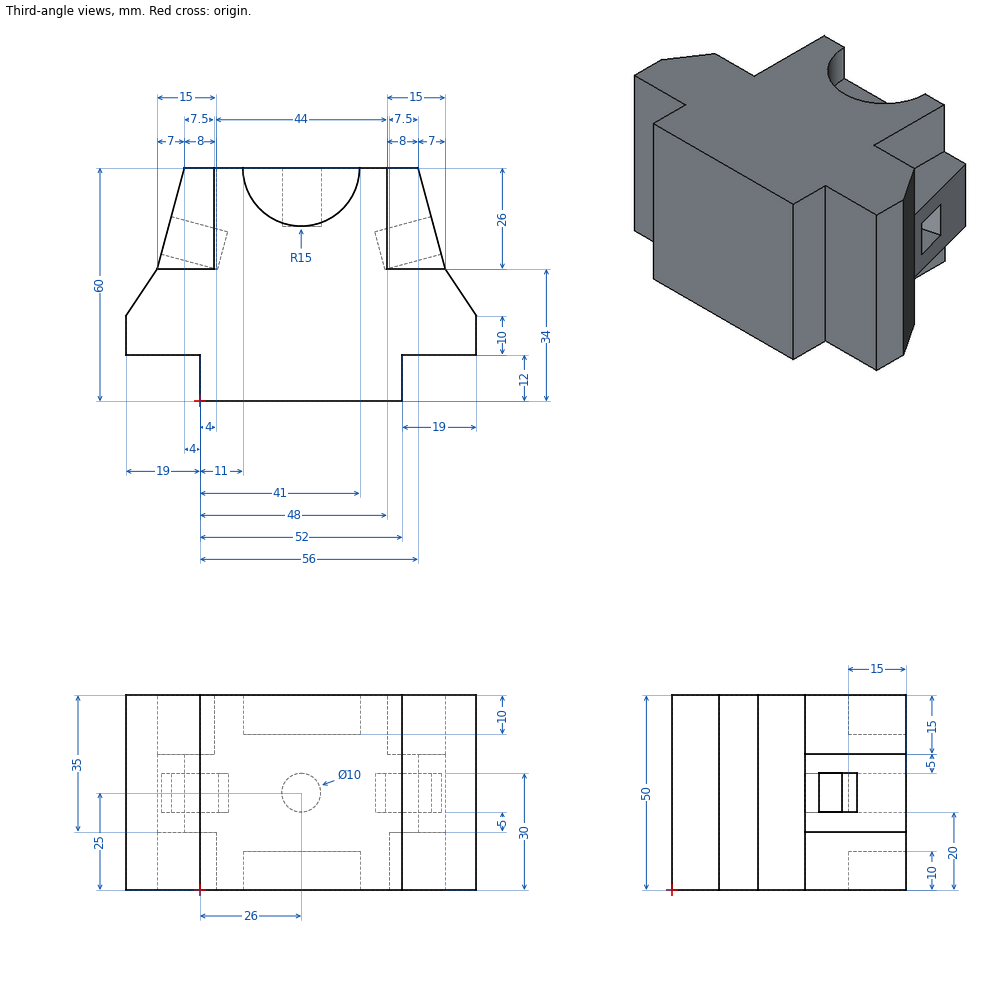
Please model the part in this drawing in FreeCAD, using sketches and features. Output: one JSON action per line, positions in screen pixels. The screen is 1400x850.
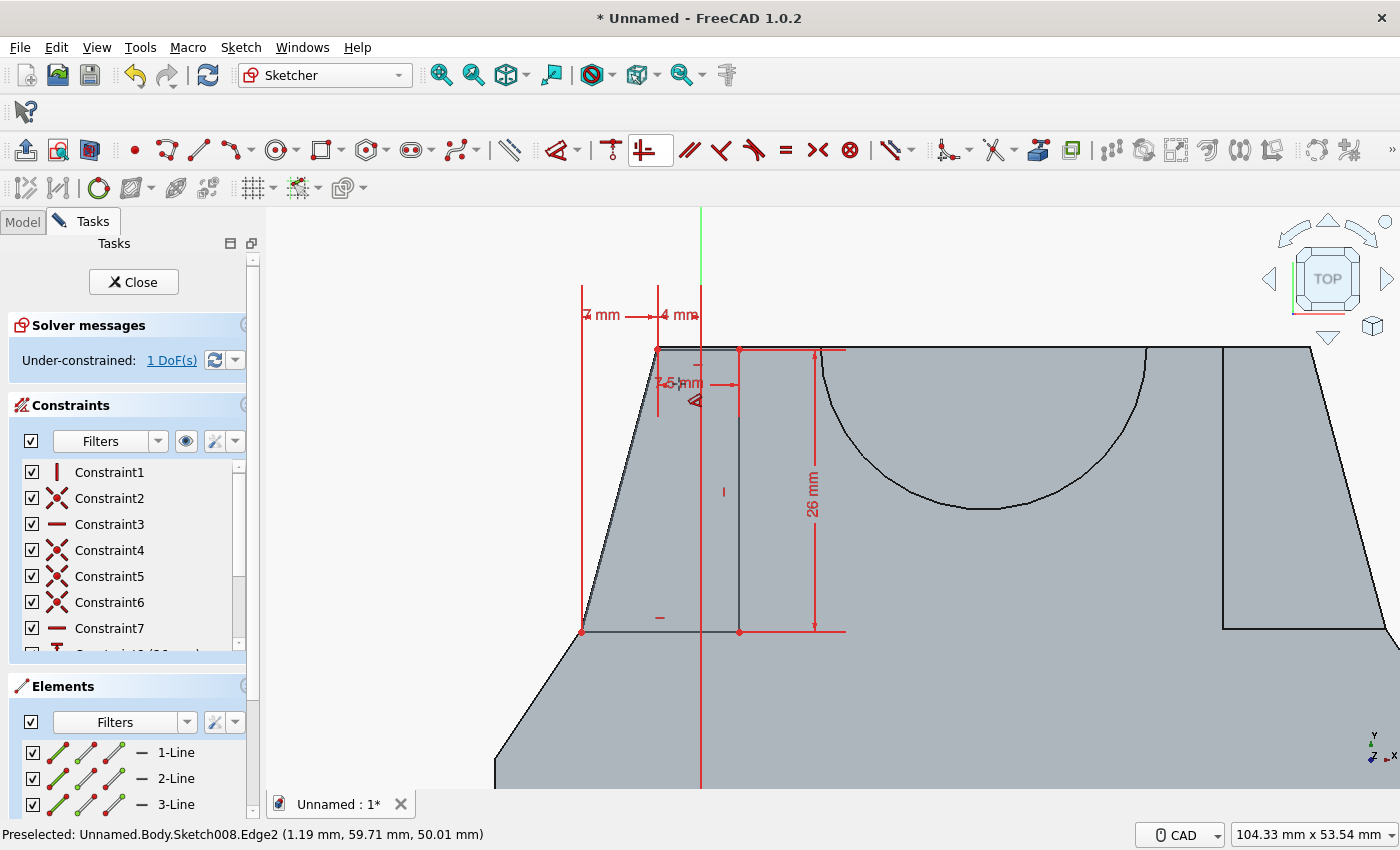
{"action": "left_click", "coordinate": [739, 632]}
{"action": "left_click", "coordinate": [773, 697]}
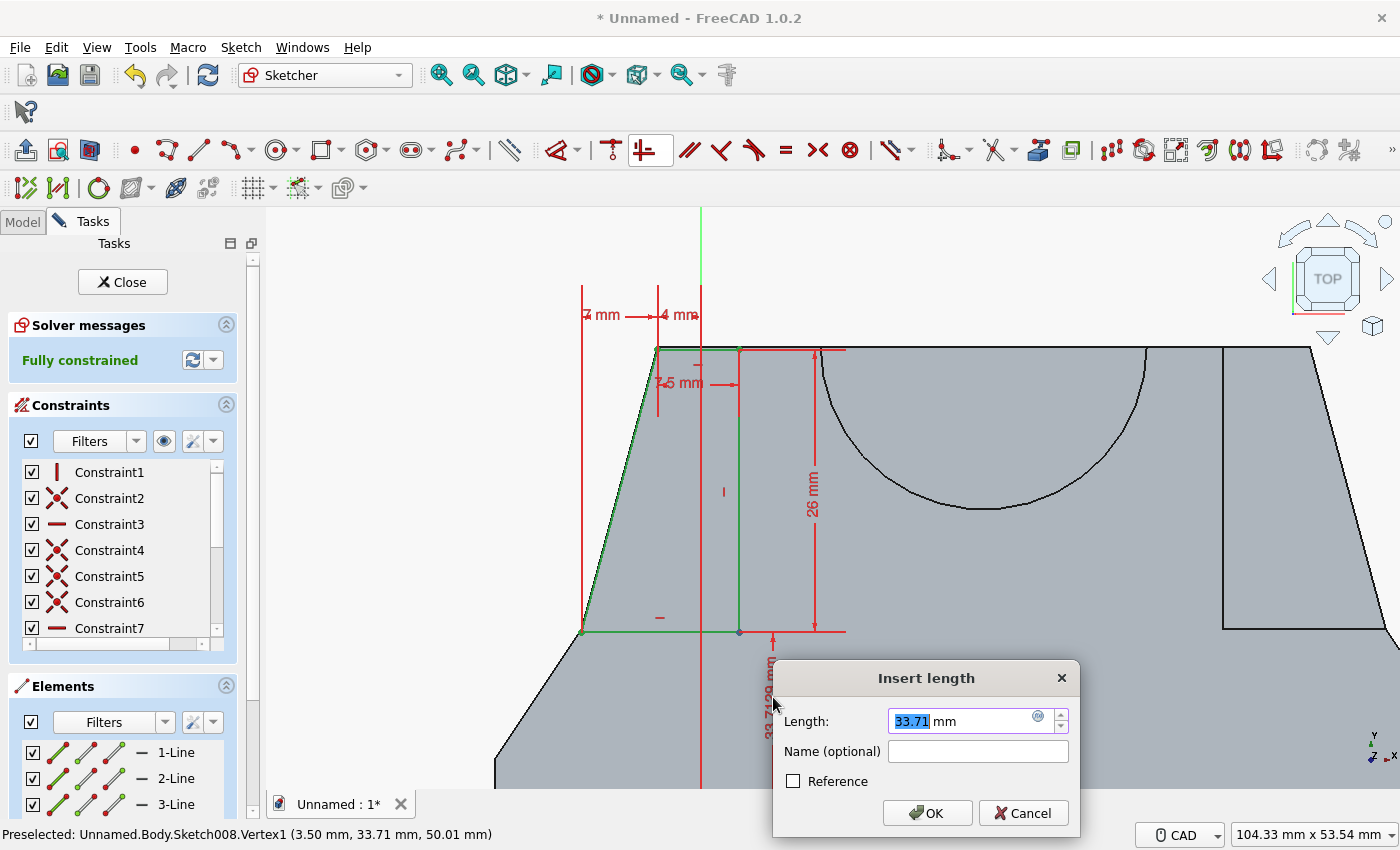
{"action": "type", "text": "34"}
{"action": "key", "text": "Return"}
{"action": "key", "text": "Escape"}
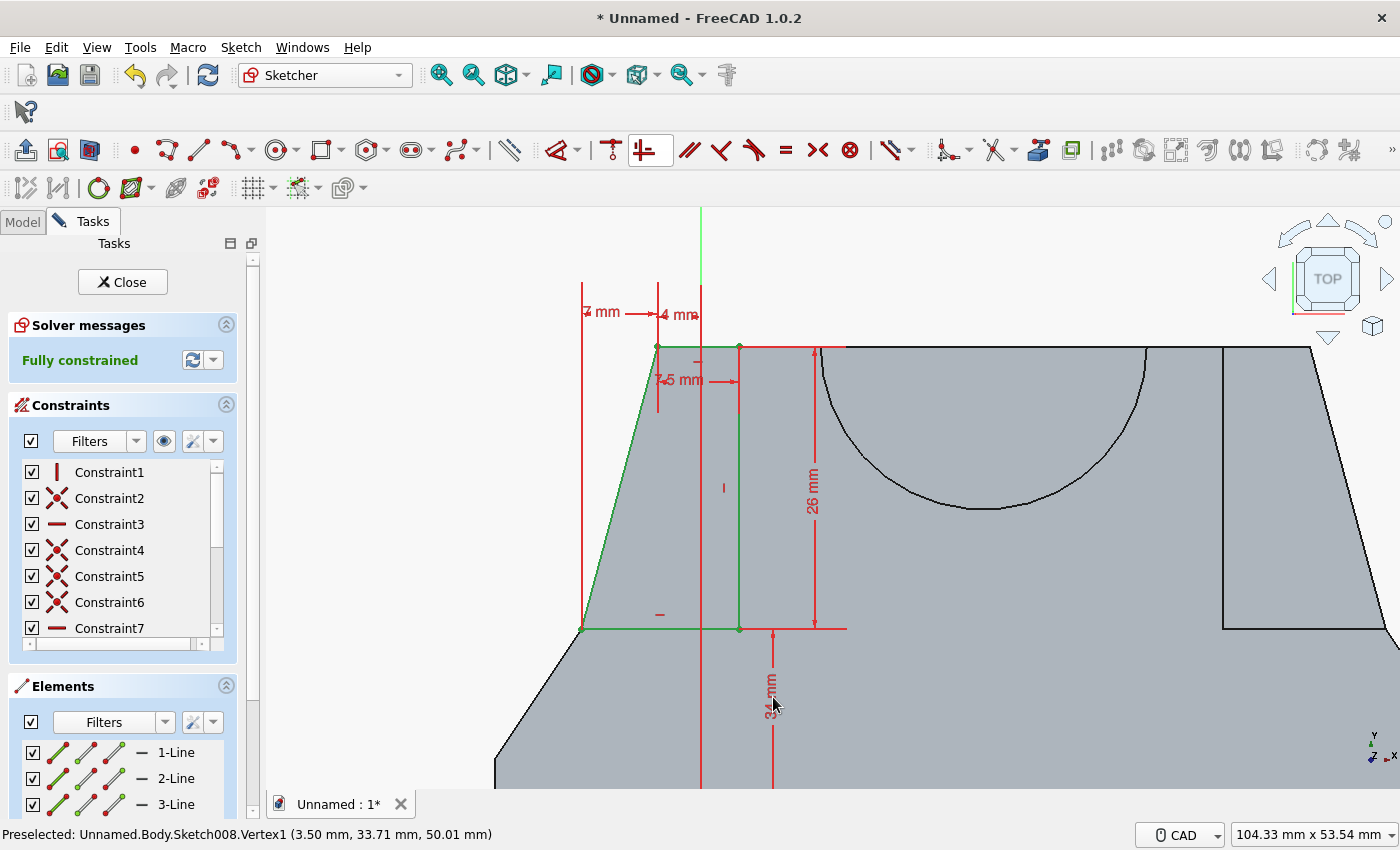
{"action": "left_click", "coordinate": [123, 282]}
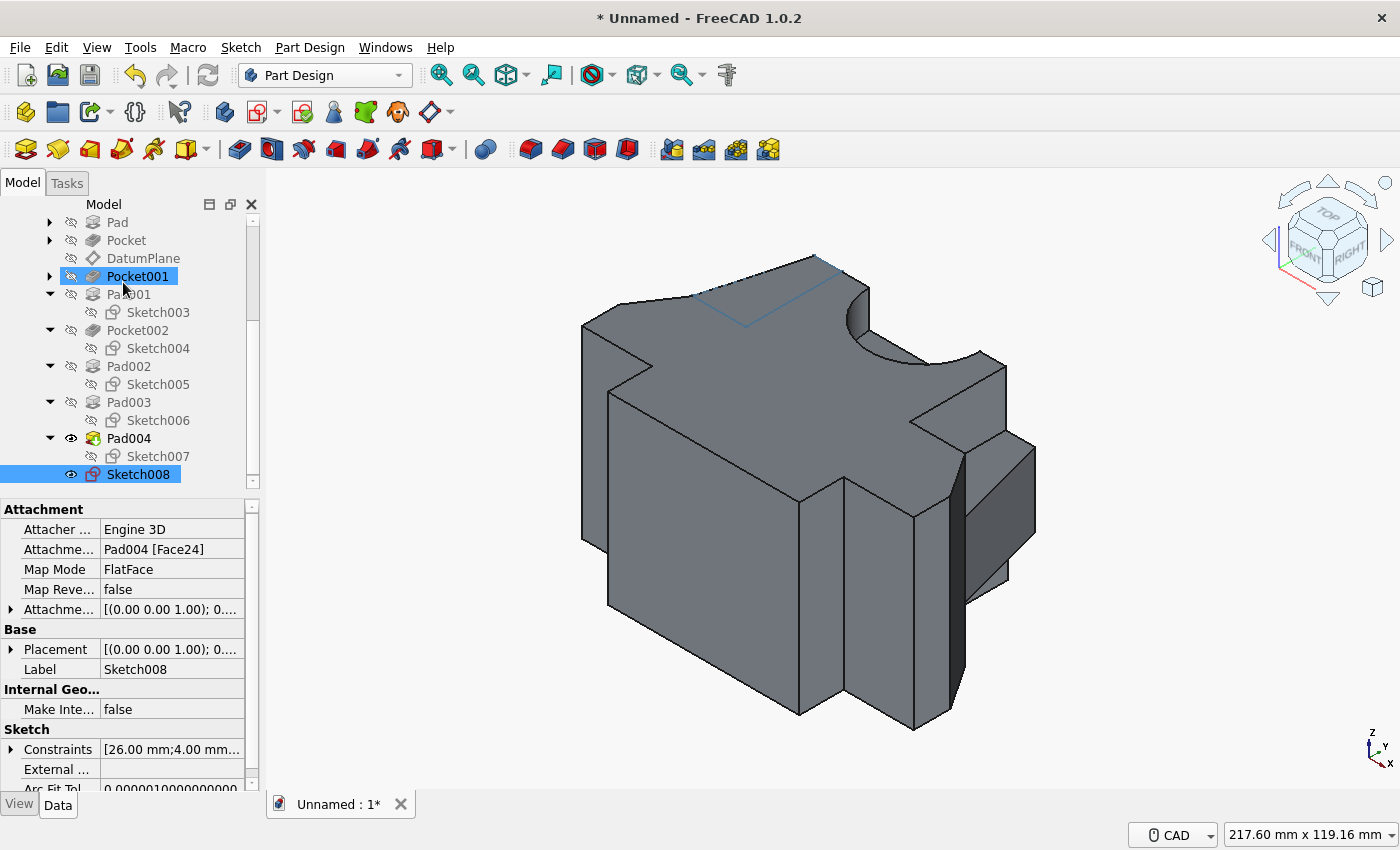
{"action": "left_click", "coordinate": [240, 150]}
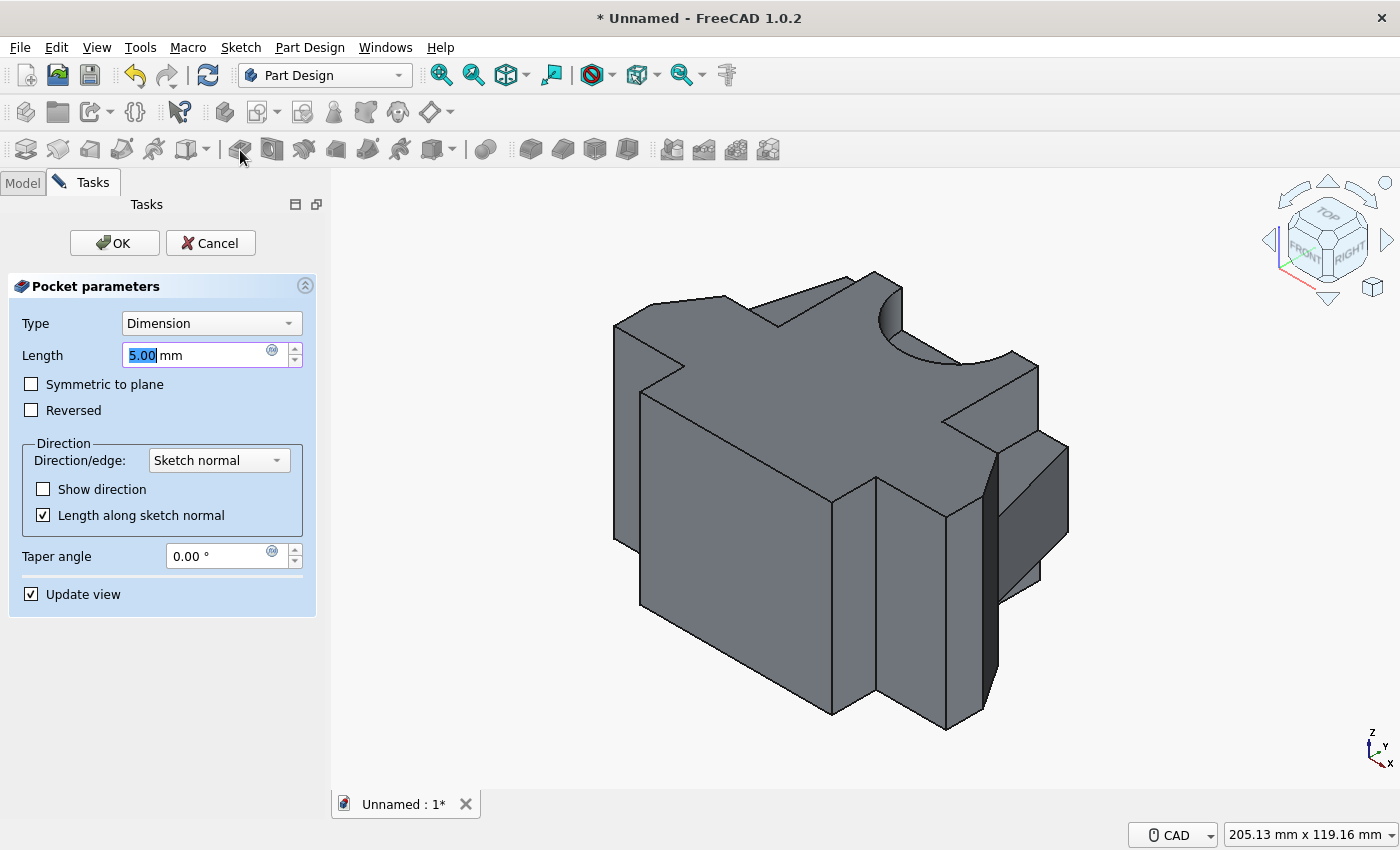
{"action": "type", "text": "15"}
{"action": "key", "text": "Tab"}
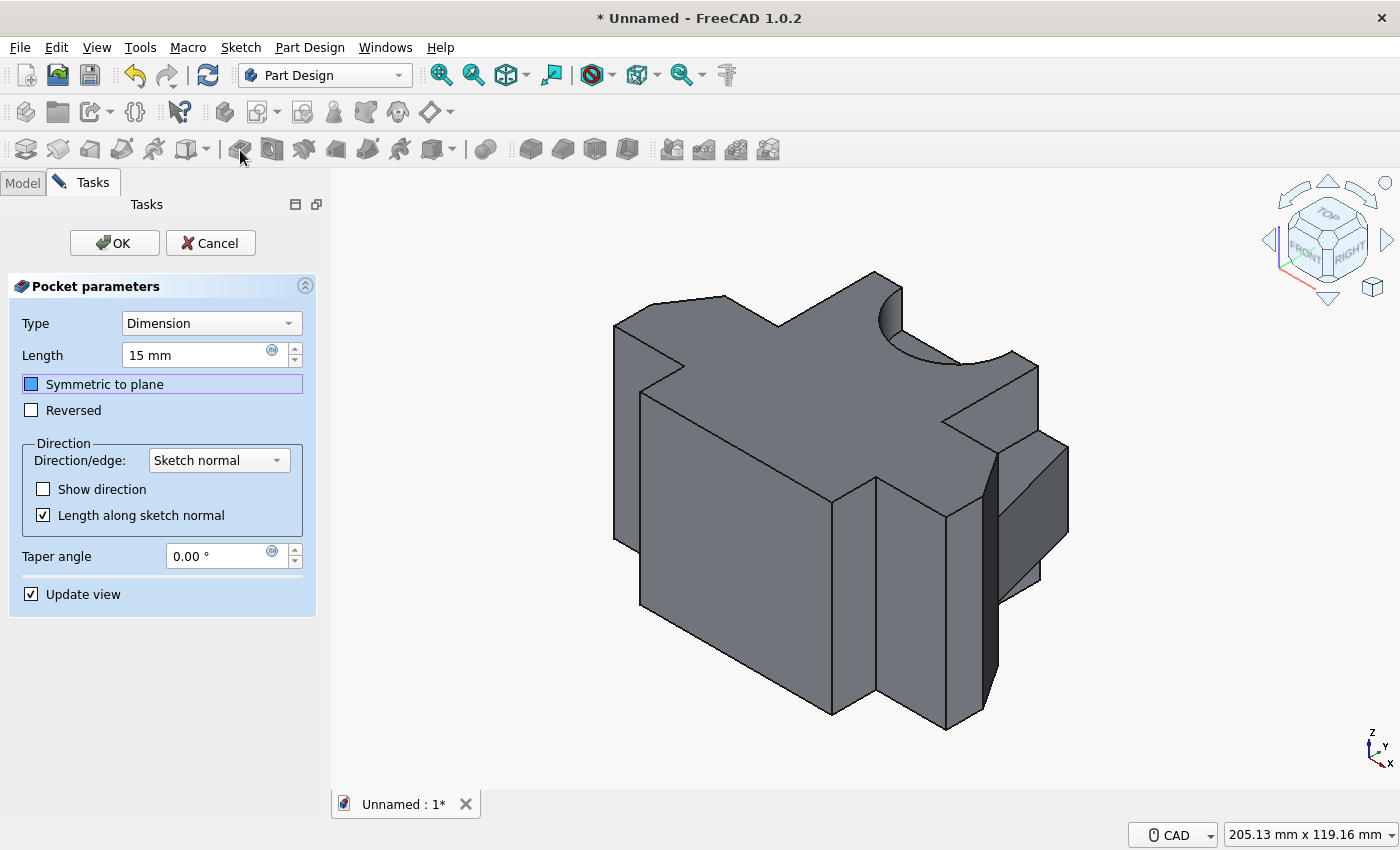
{"action": "left_click", "coordinate": [115, 243]}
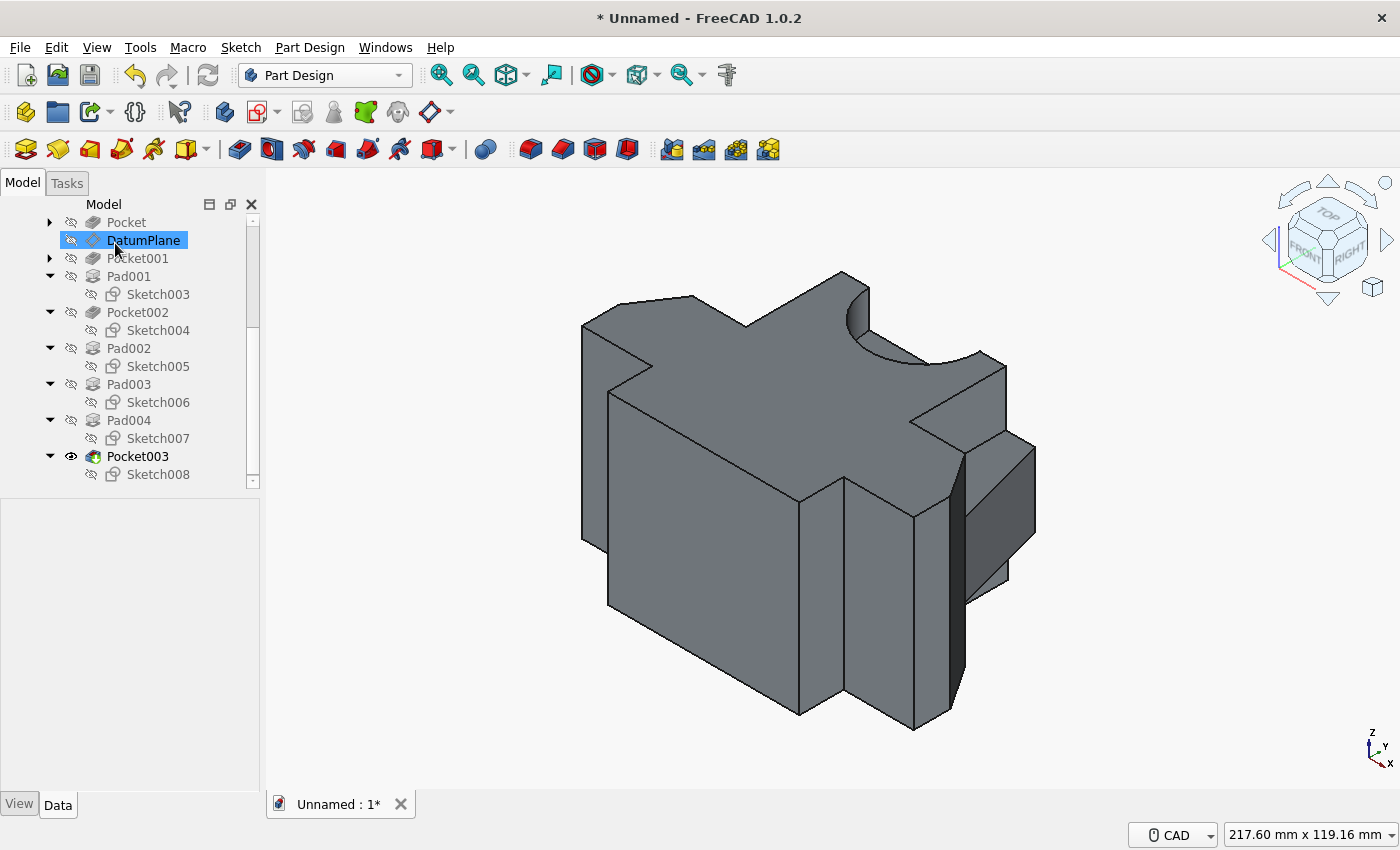
{"action": "key", "text": "4"}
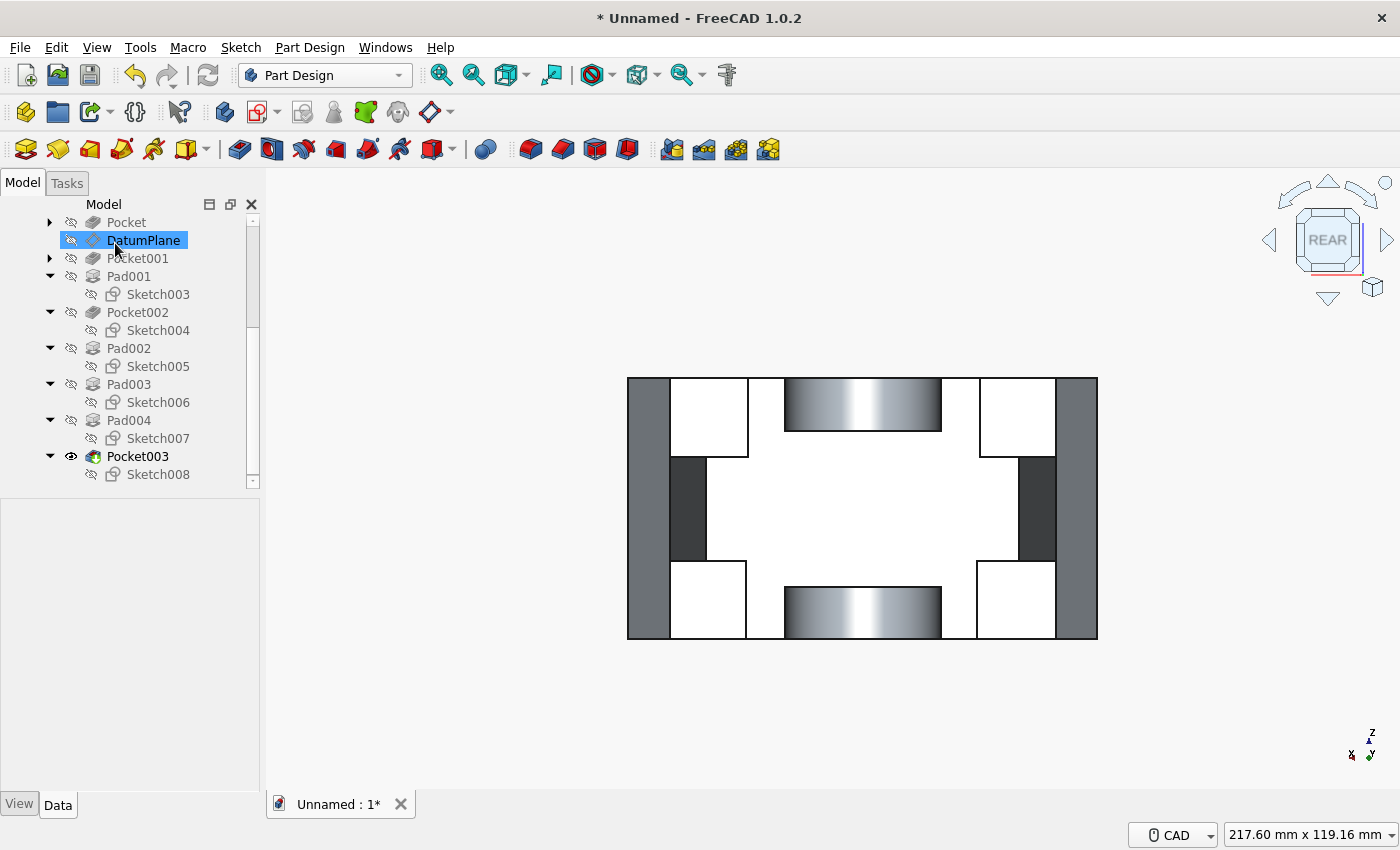
{"action": "left_click", "coordinate": [442, 76]}